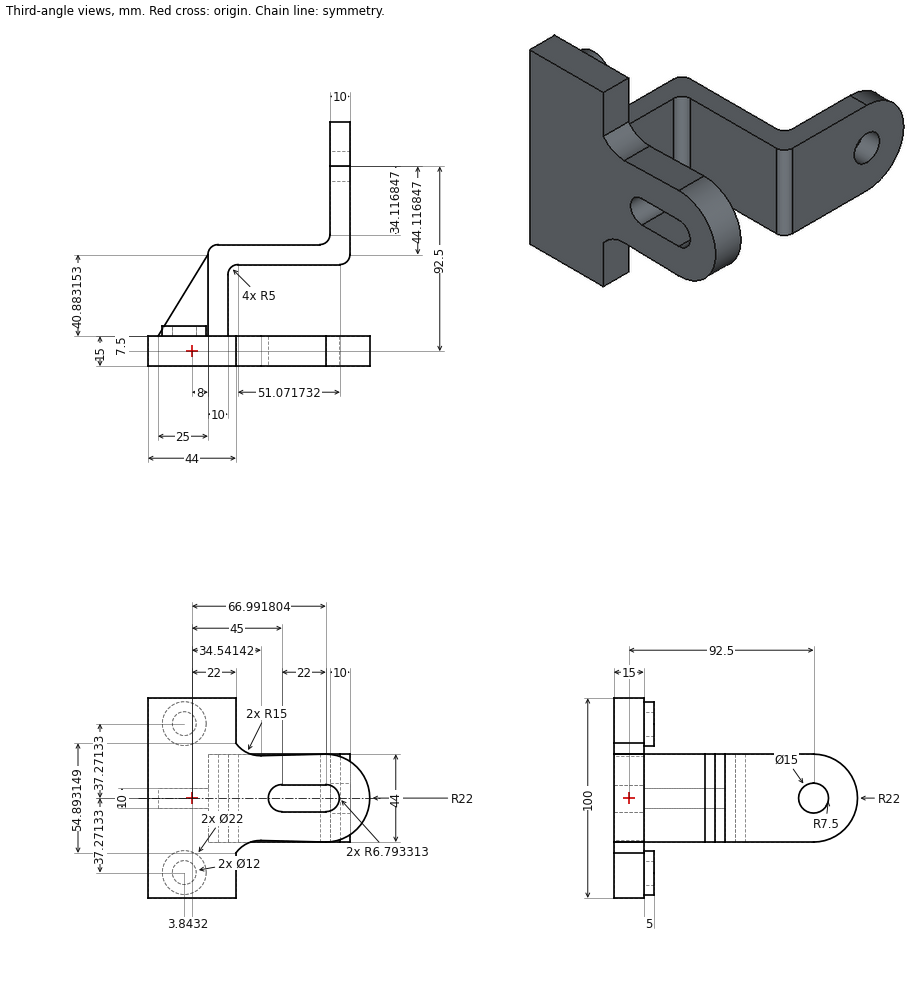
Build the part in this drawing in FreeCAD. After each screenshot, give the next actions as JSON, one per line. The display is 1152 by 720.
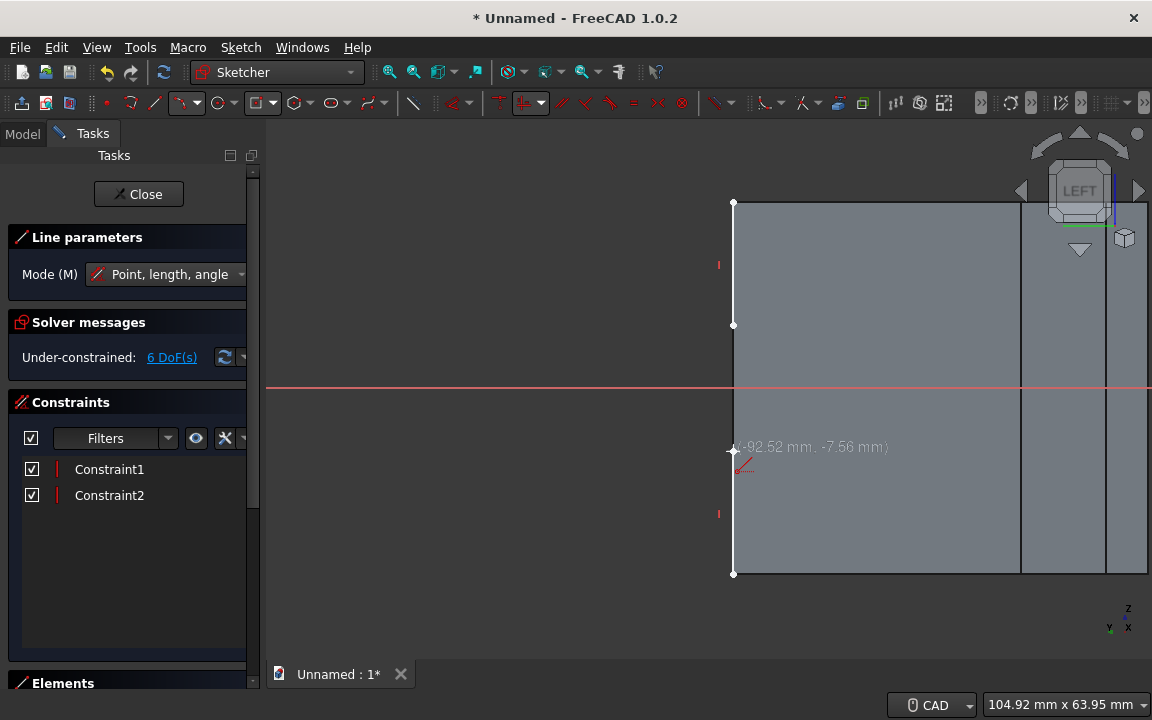
{"action": "left_click", "coordinate": [180, 104]}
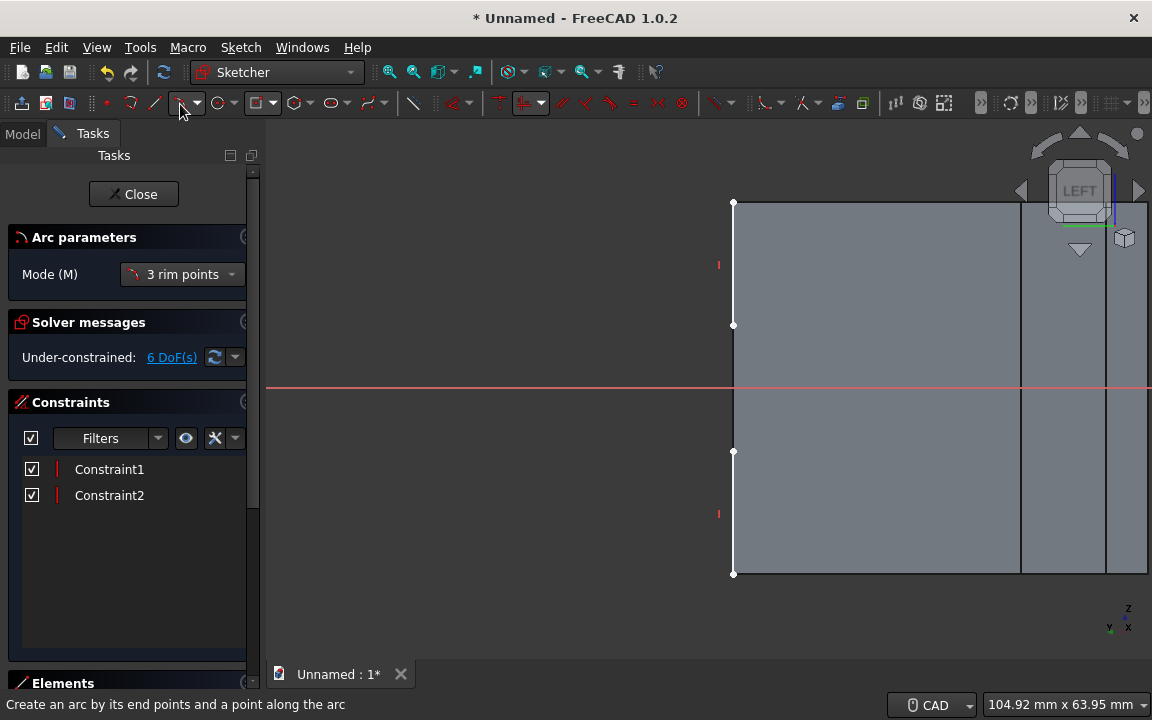
{"action": "left_click", "coordinate": [733, 203]}
{"action": "left_click", "coordinate": [733, 575]}
{"action": "left_click", "coordinate": [556, 331]}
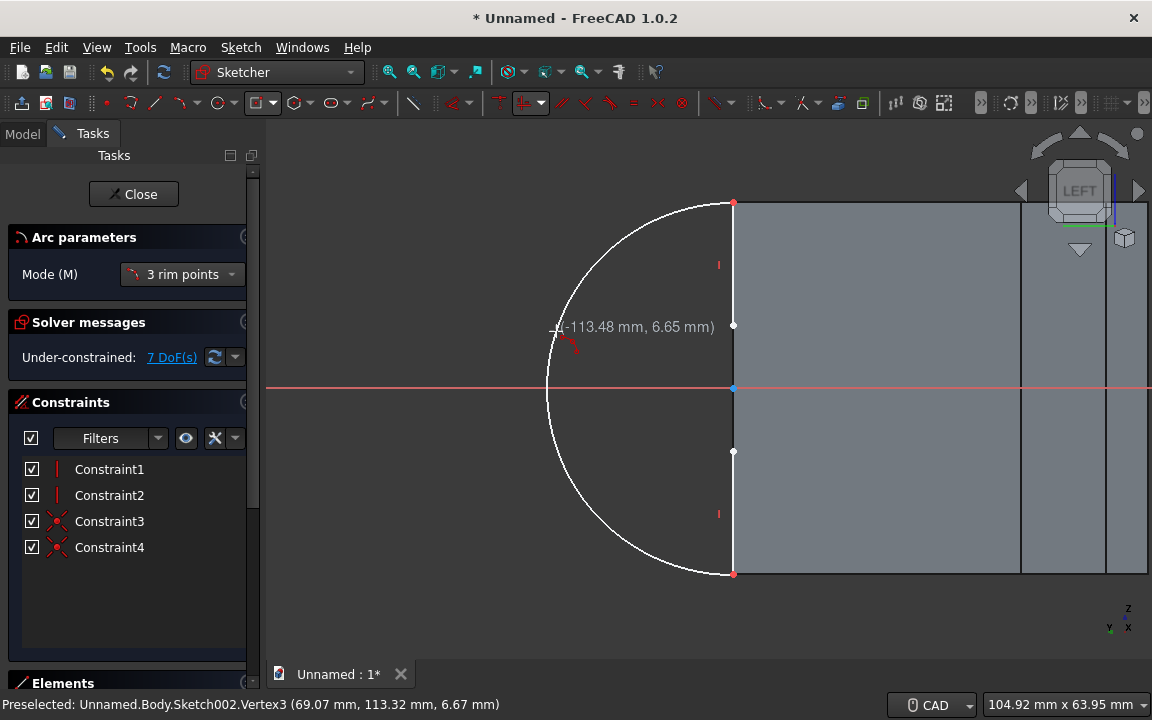
{"action": "left_click", "coordinate": [733, 452]}
{"action": "left_click", "coordinate": [733, 326]}
{"action": "left_click", "coordinate": [673, 369]}
{"action": "key", "text": "Escape"}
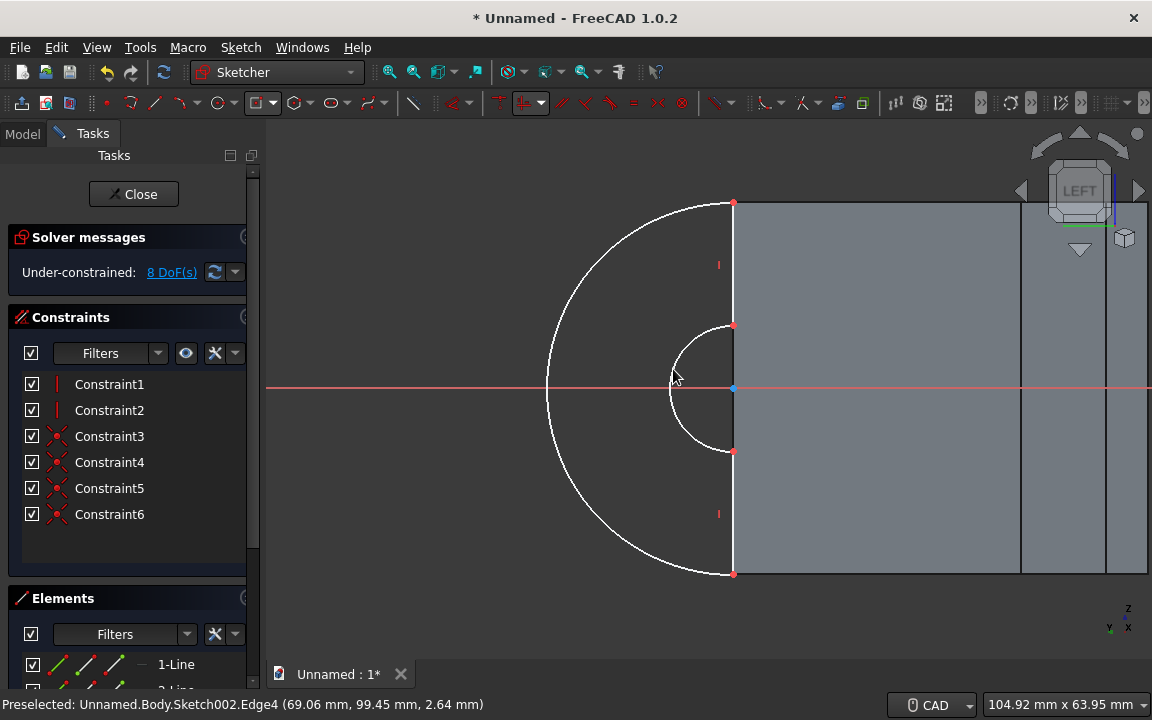
{"action": "left_click", "coordinate": [583, 280]}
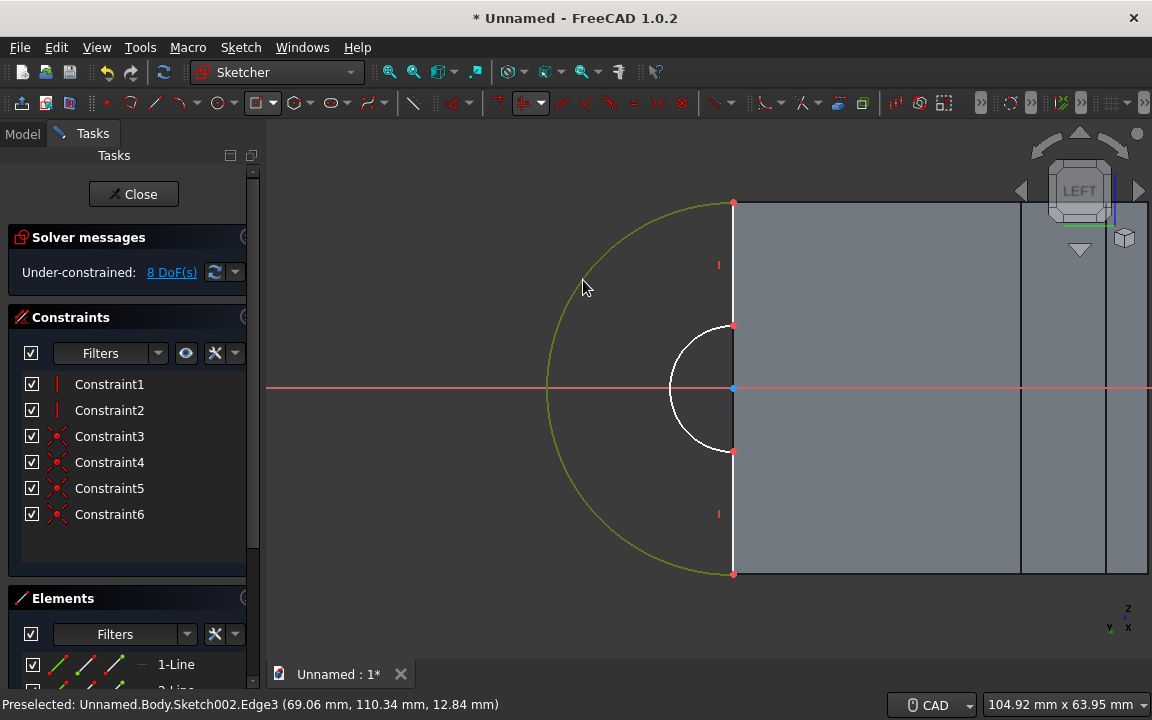
{"action": "left_click", "coordinate": [682, 352]}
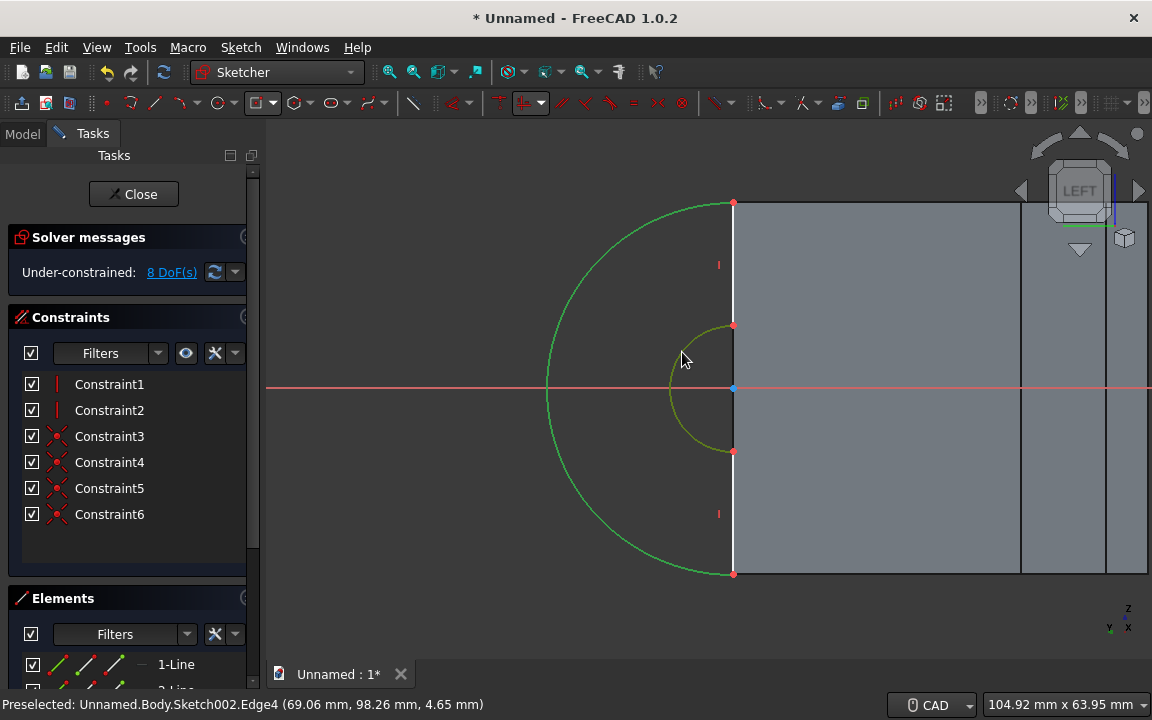
{"action": "left_click", "coordinate": [500, 104]}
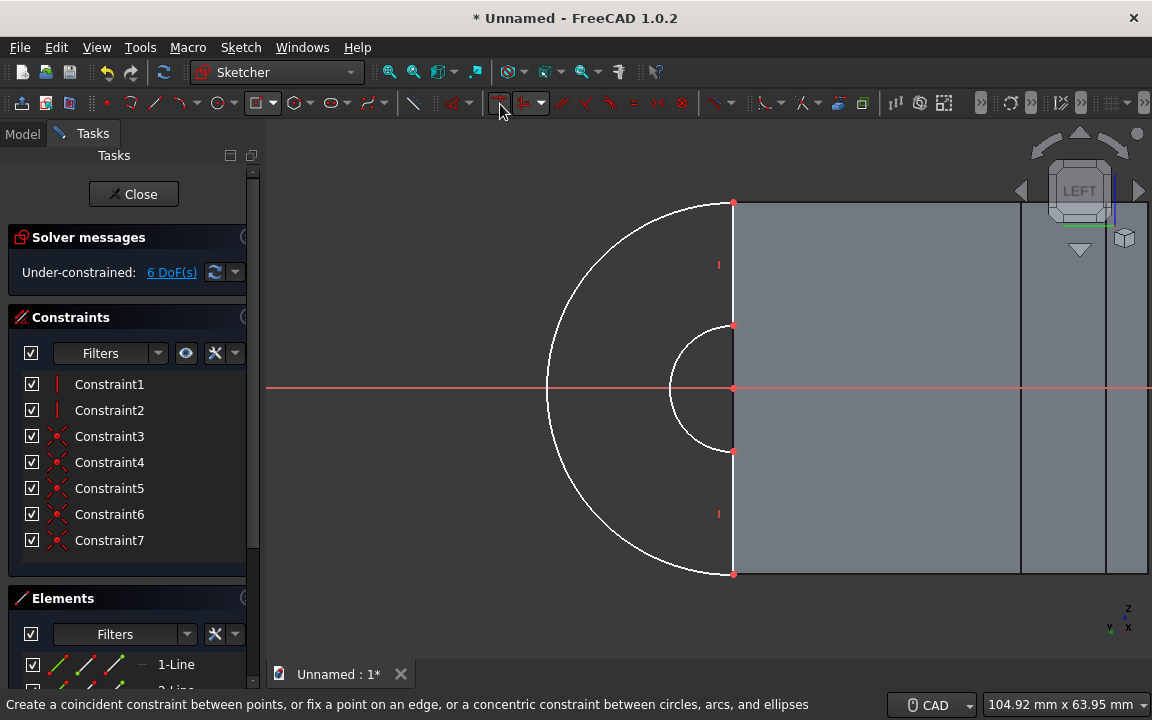
{"action": "left_click", "coordinate": [733, 389]}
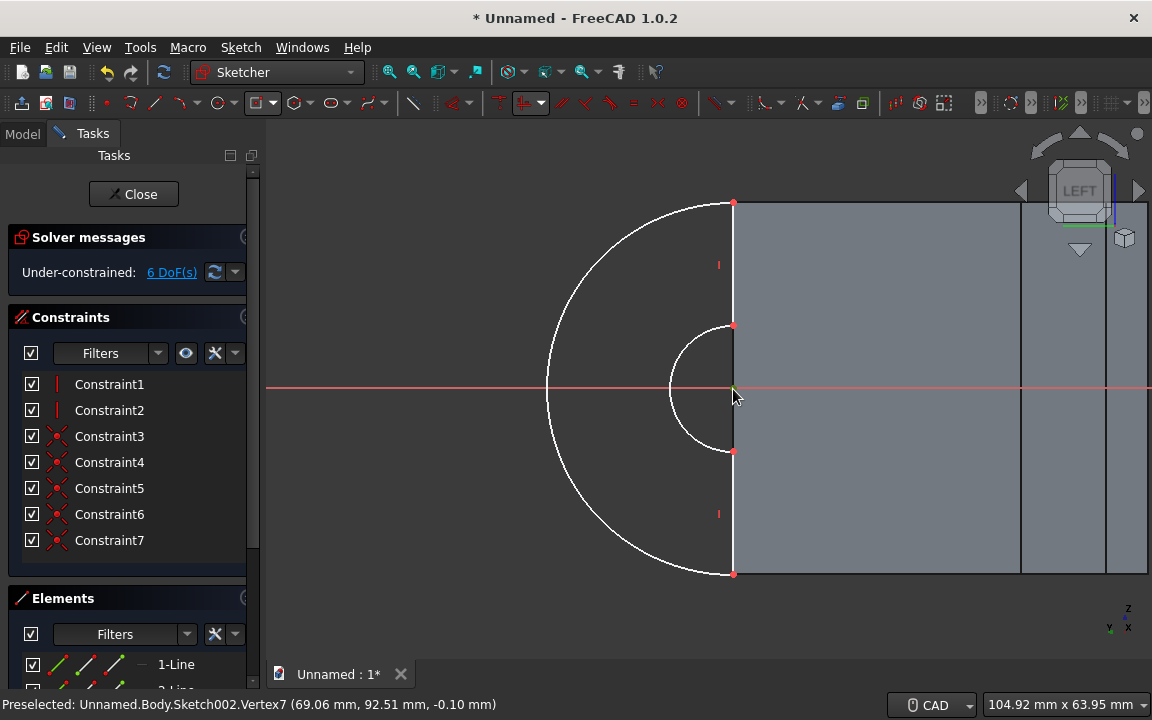
{"action": "left_click", "coordinate": [344, 388]}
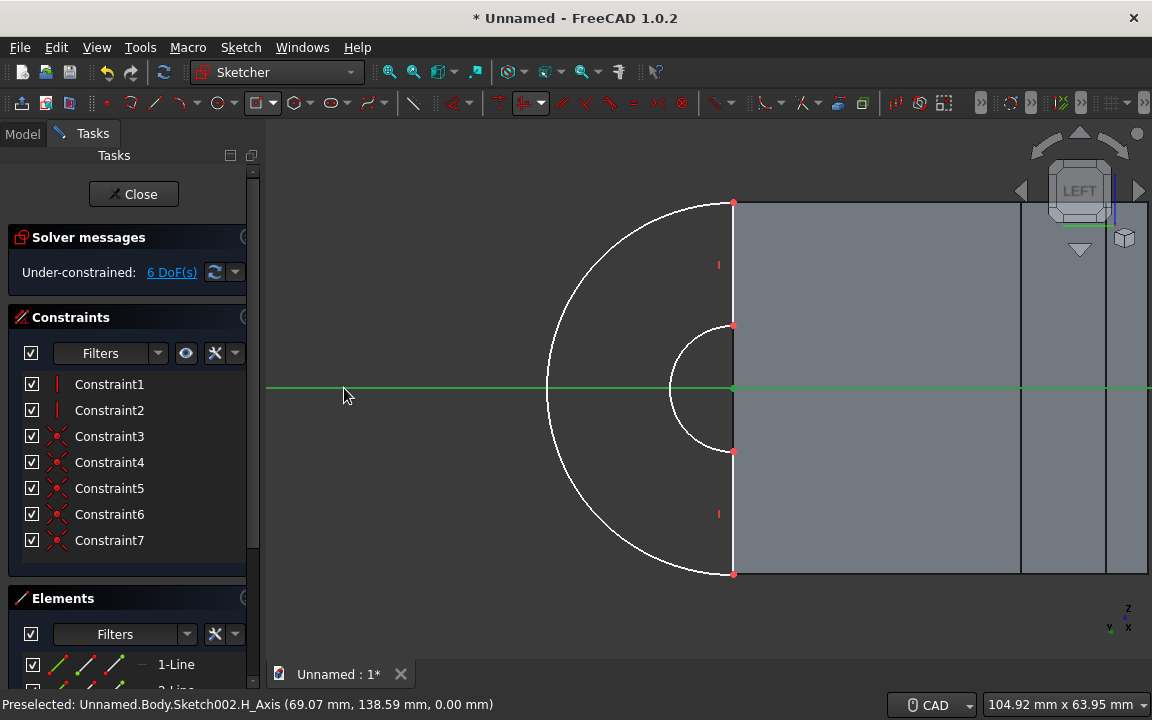
{"action": "left_click", "coordinate": [500, 104]}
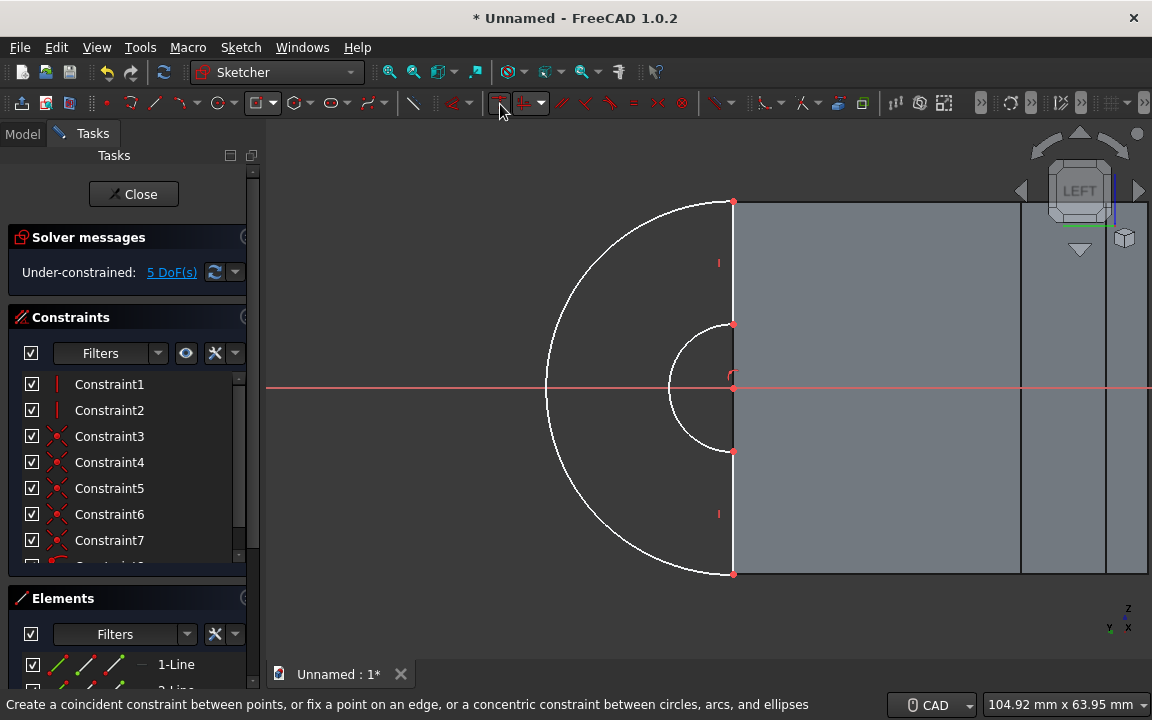
{"action": "left_click", "coordinate": [452, 104]}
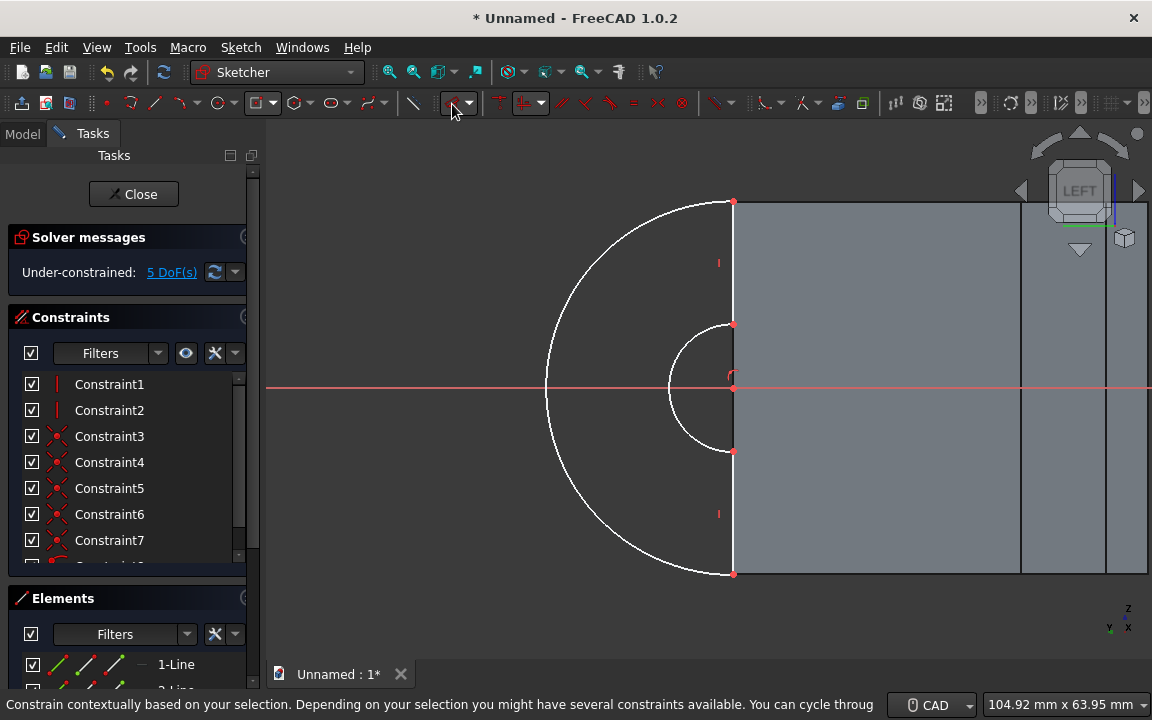
{"action": "left_click", "coordinate": [582, 278]}
{"action": "left_click", "coordinate": [556, 259]}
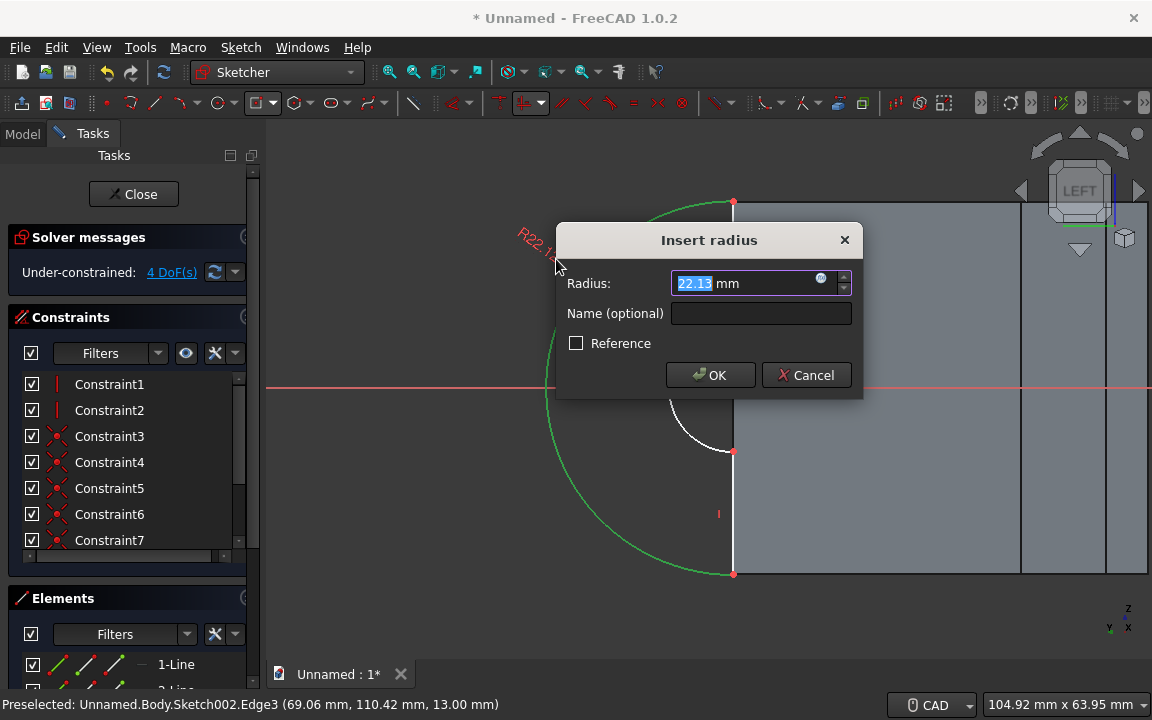
{"action": "type", "text": "22"}
{"action": "key", "text": "Return"}